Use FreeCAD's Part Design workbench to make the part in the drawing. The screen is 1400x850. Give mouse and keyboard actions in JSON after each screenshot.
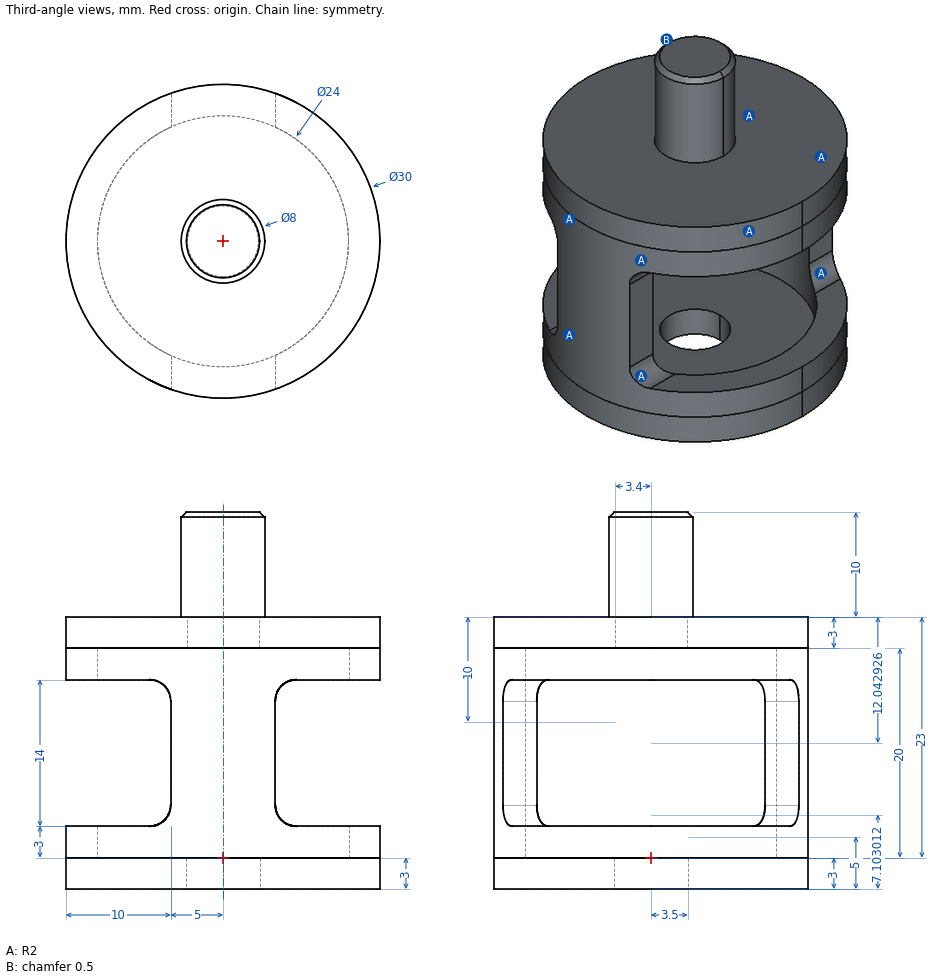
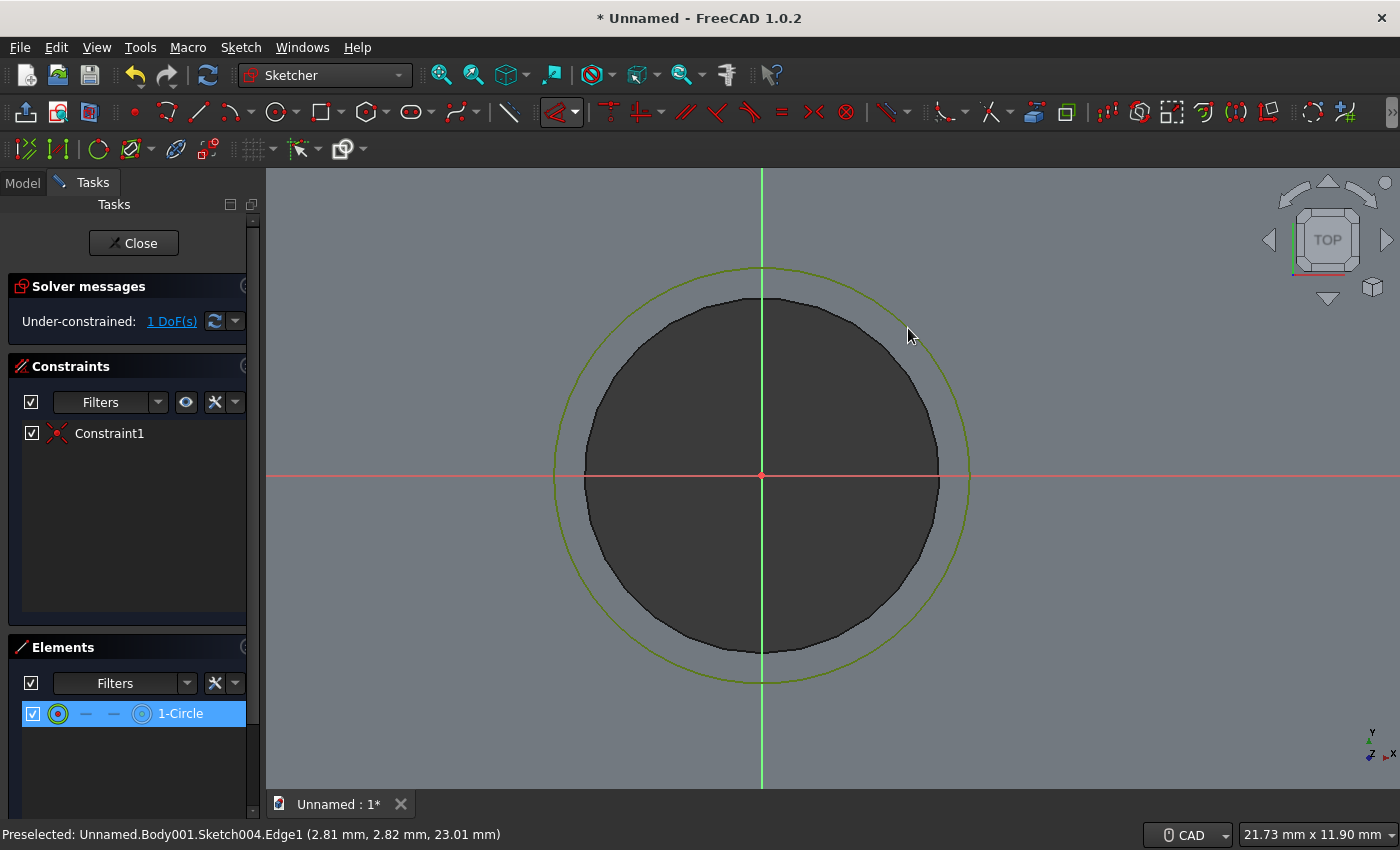
{"action": "key", "text": "k o"}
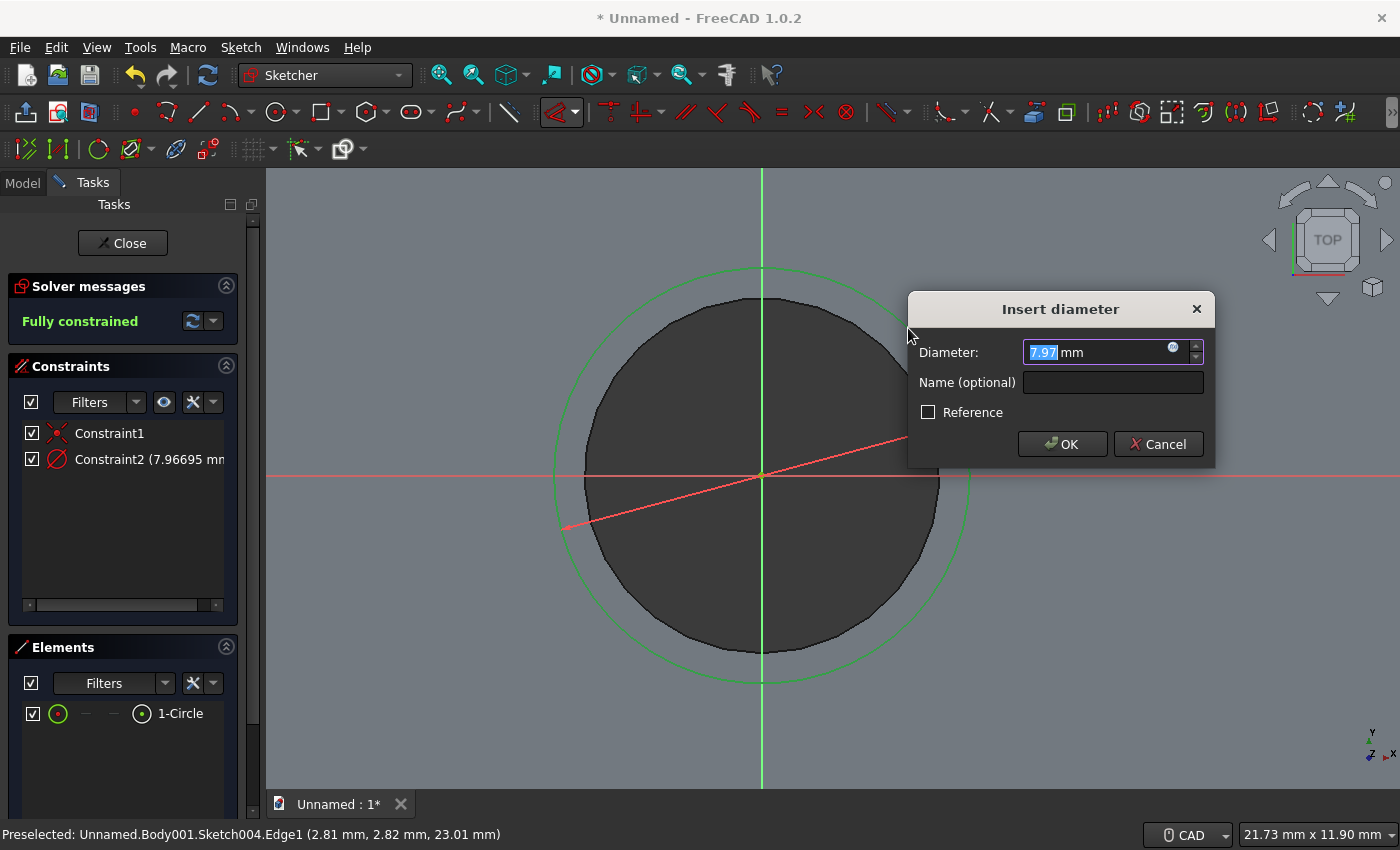
{"action": "type", "text": "8"}
{"action": "key", "text": "Return"}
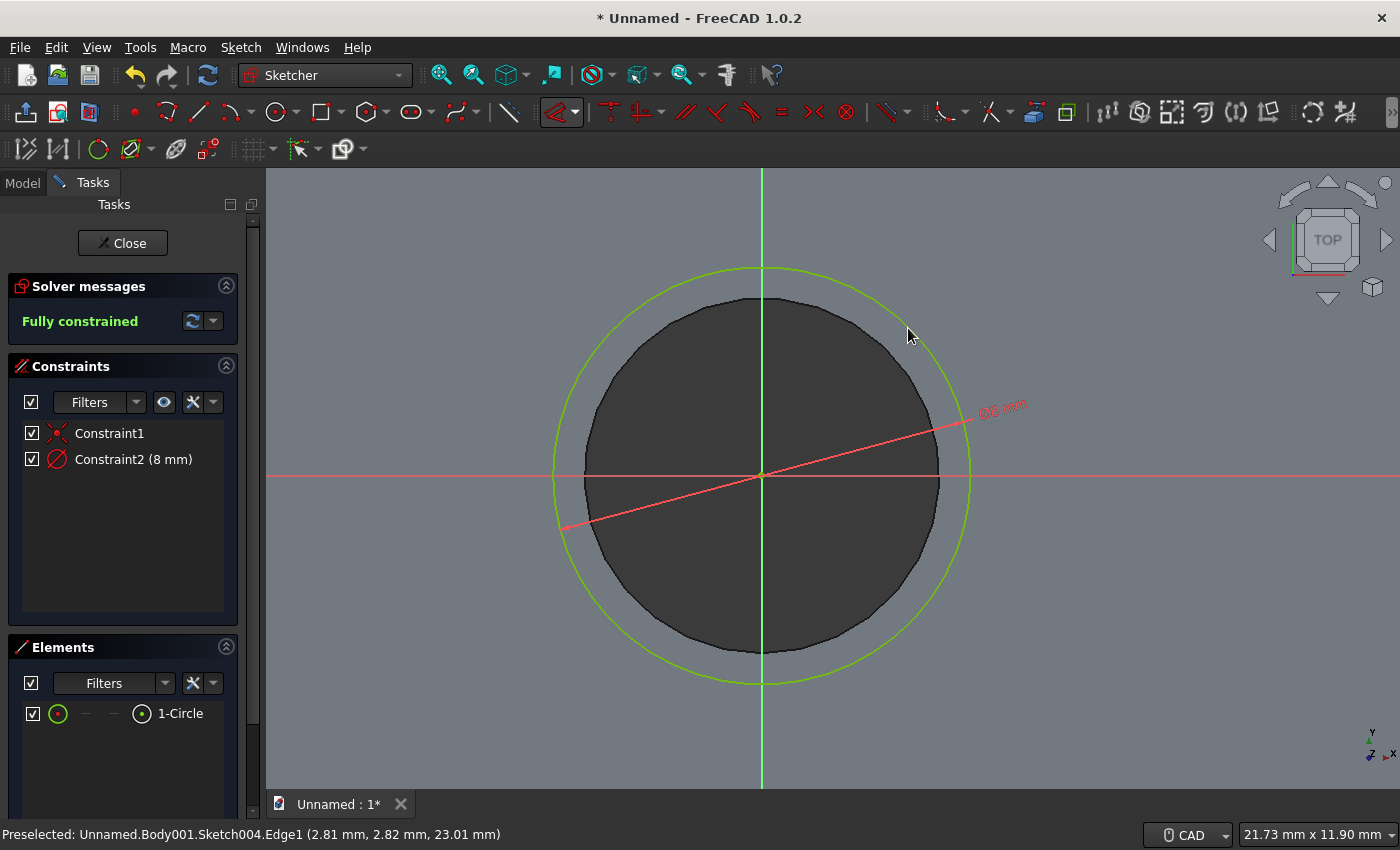
{"action": "left_click", "coordinate": [123, 243]}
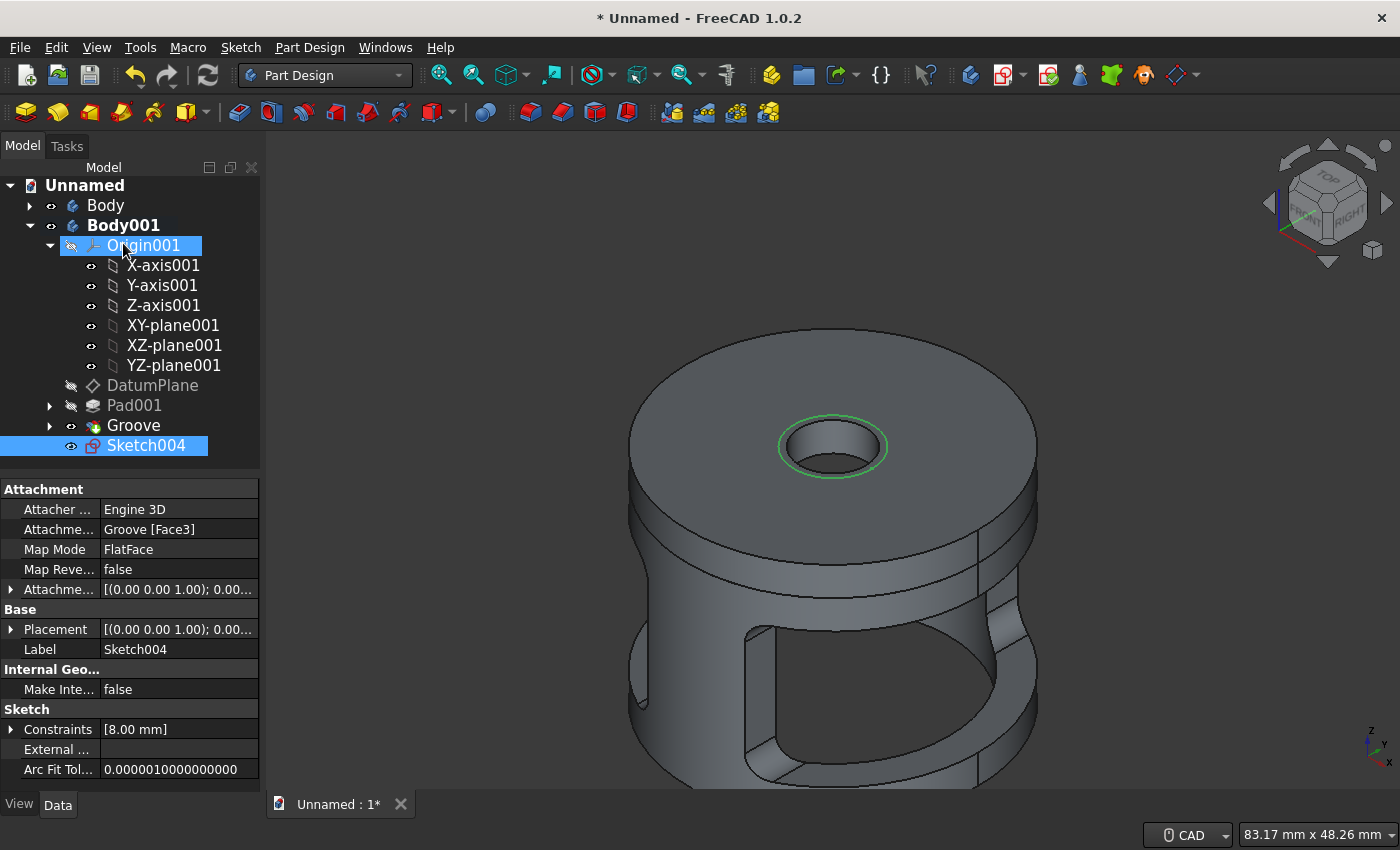
{"action": "left_click", "coordinate": [26, 112]}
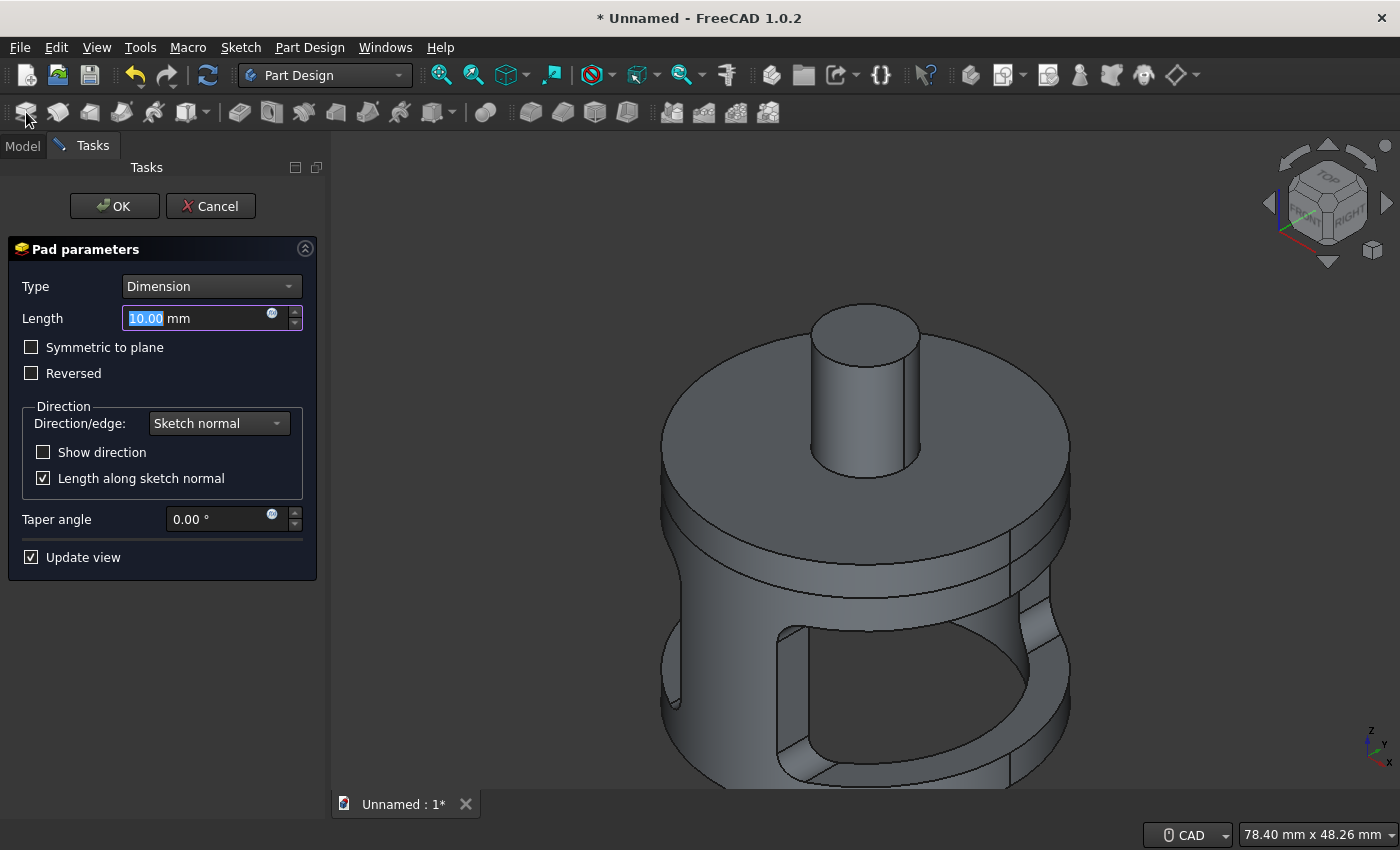
{"action": "type", "text": "10"}
{"action": "key", "text": "Tab"}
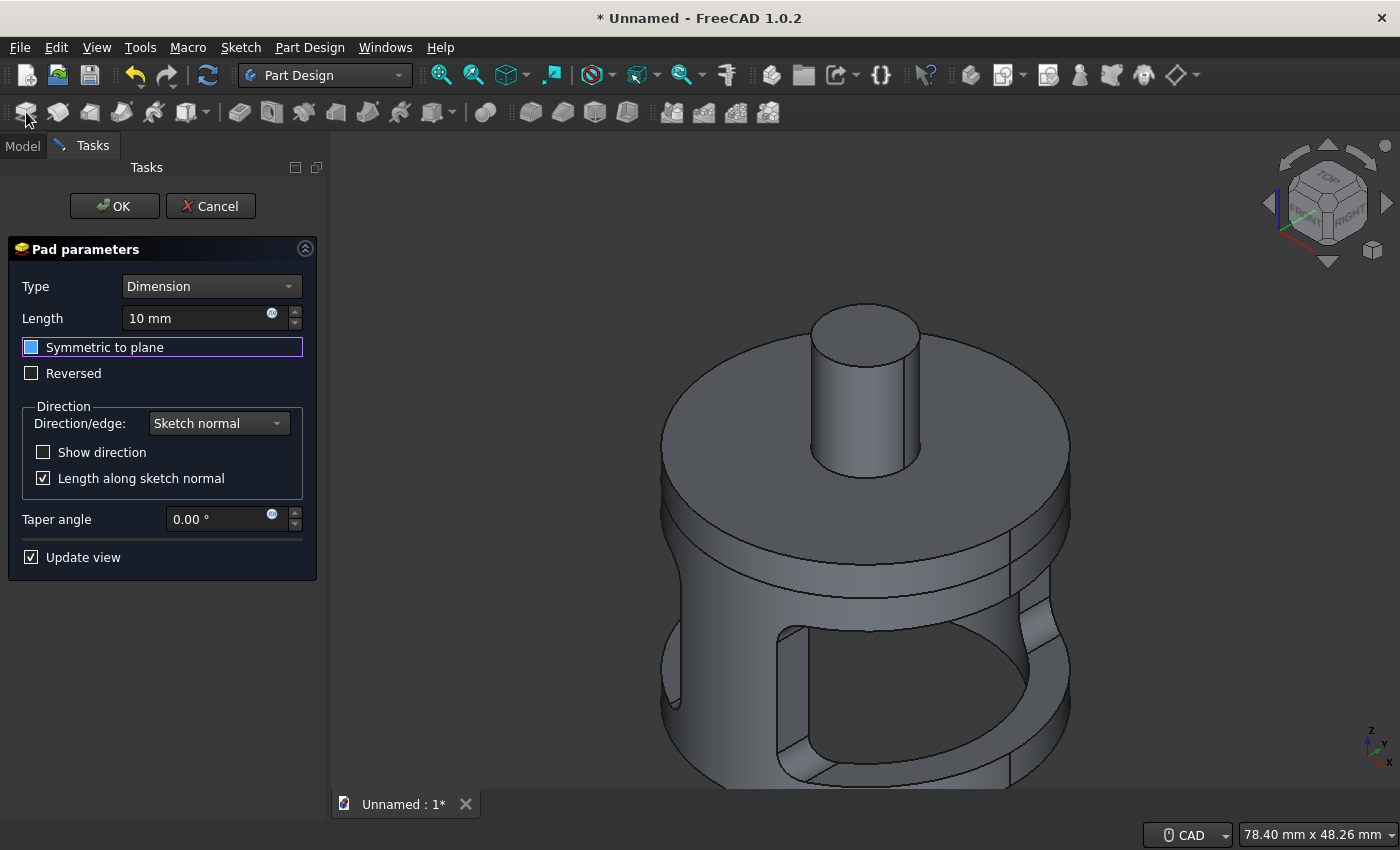
{"action": "left_click", "coordinate": [115, 206]}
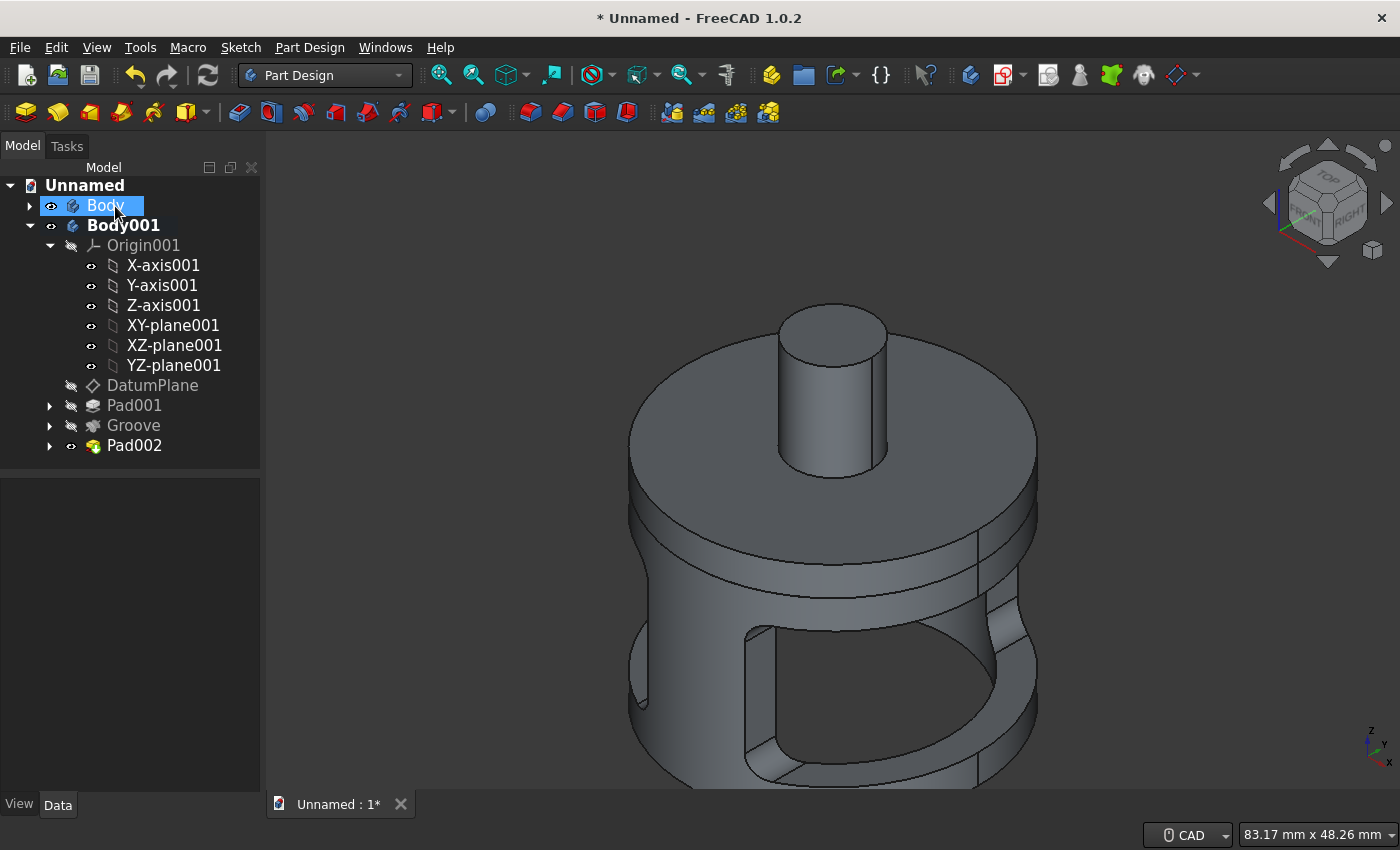
{"action": "left_click", "coordinate": [784, 349]}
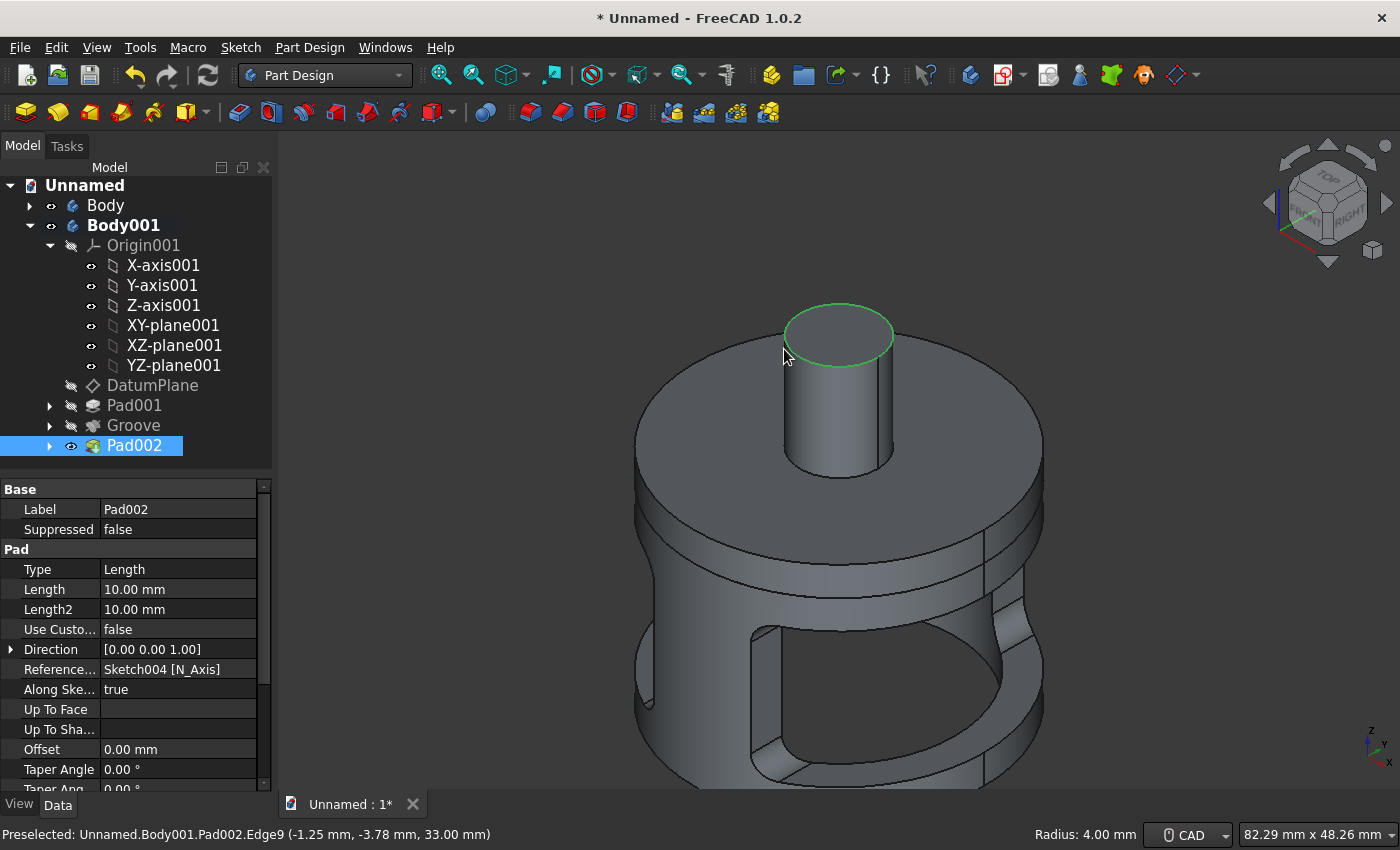
{"action": "left_click", "coordinate": [564, 112]}